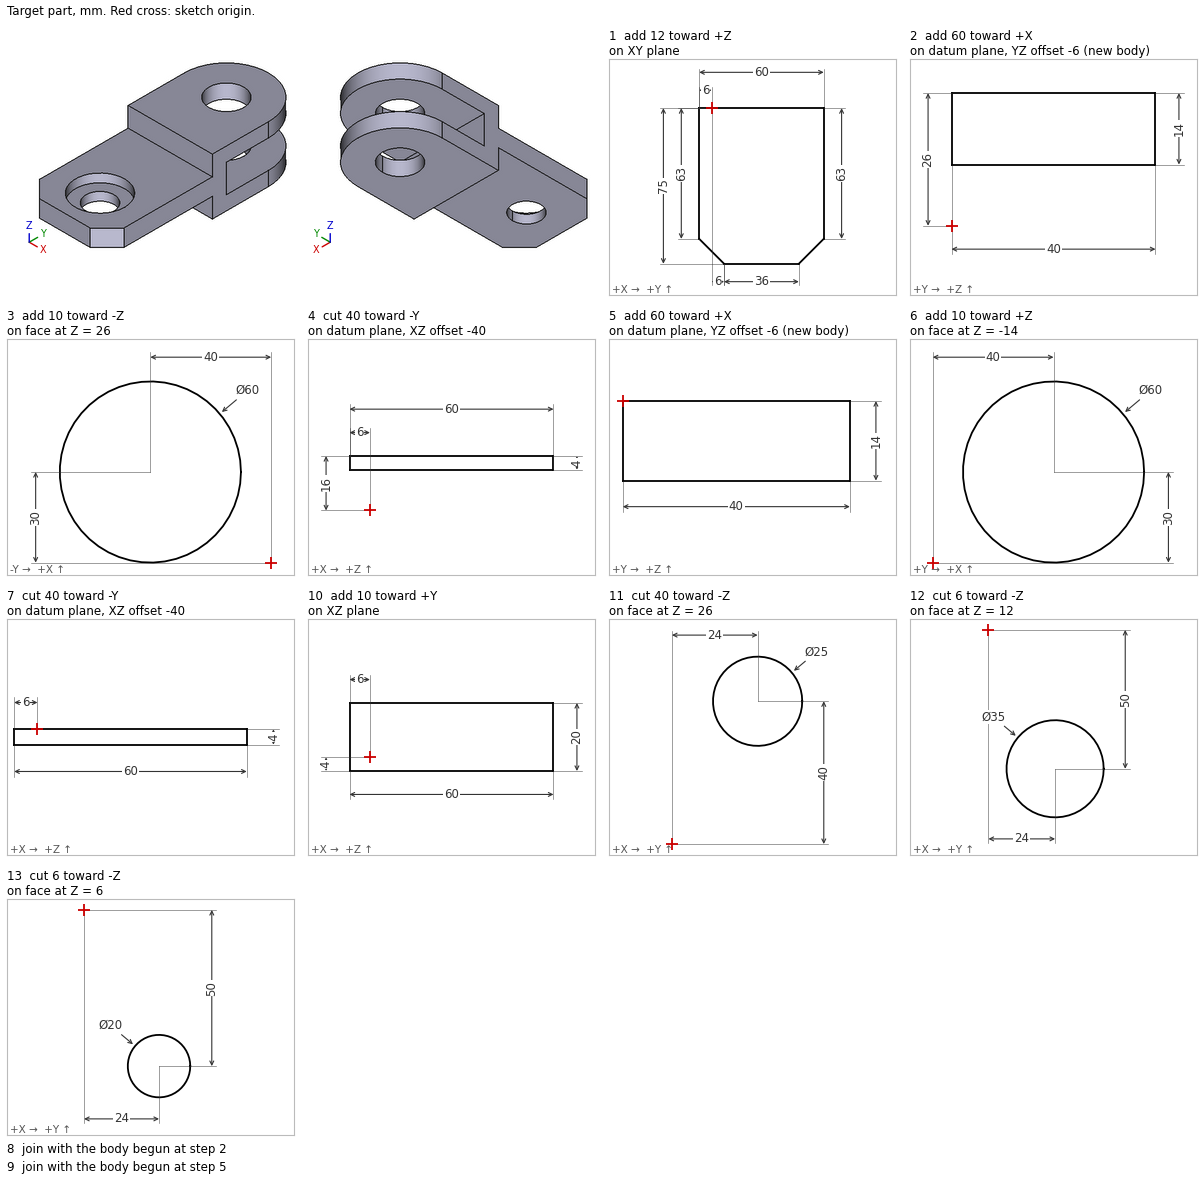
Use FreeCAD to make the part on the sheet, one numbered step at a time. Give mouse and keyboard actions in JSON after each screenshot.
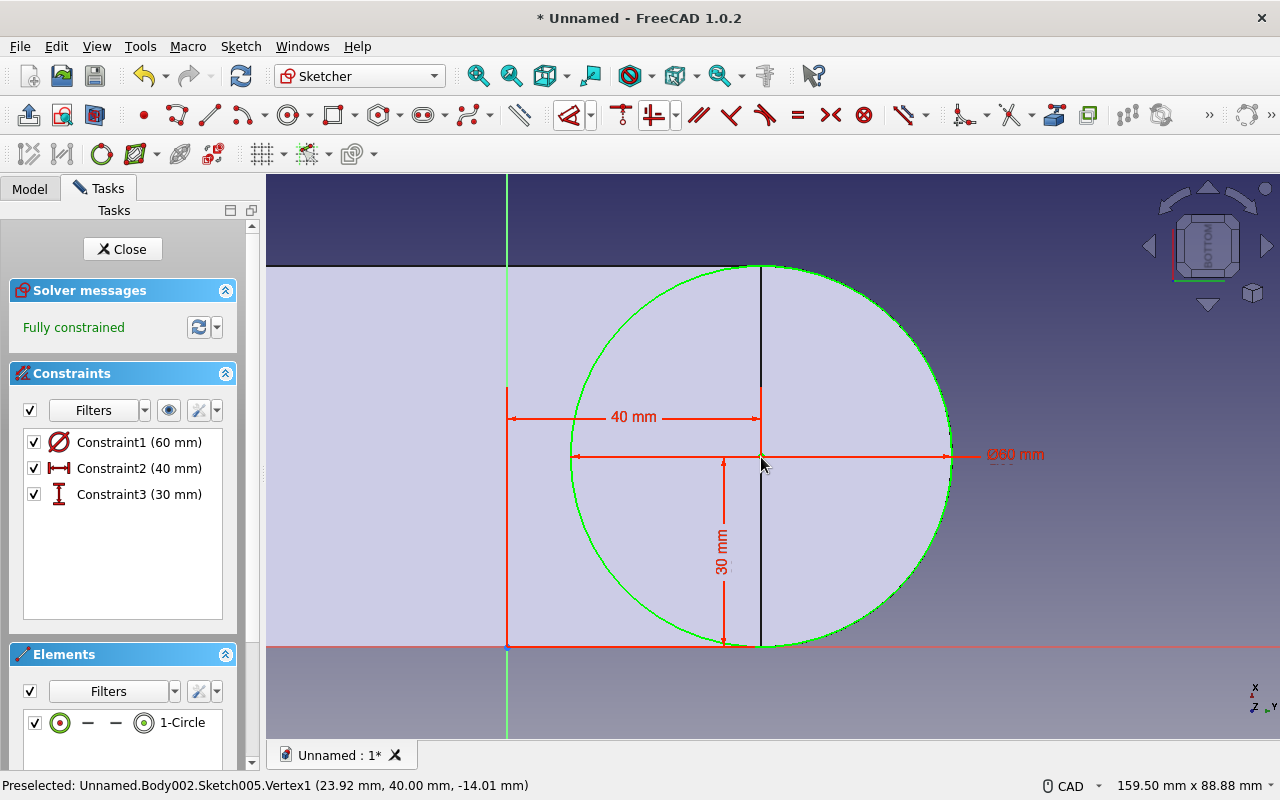
{"action": "left_click", "coordinate": [123, 249]}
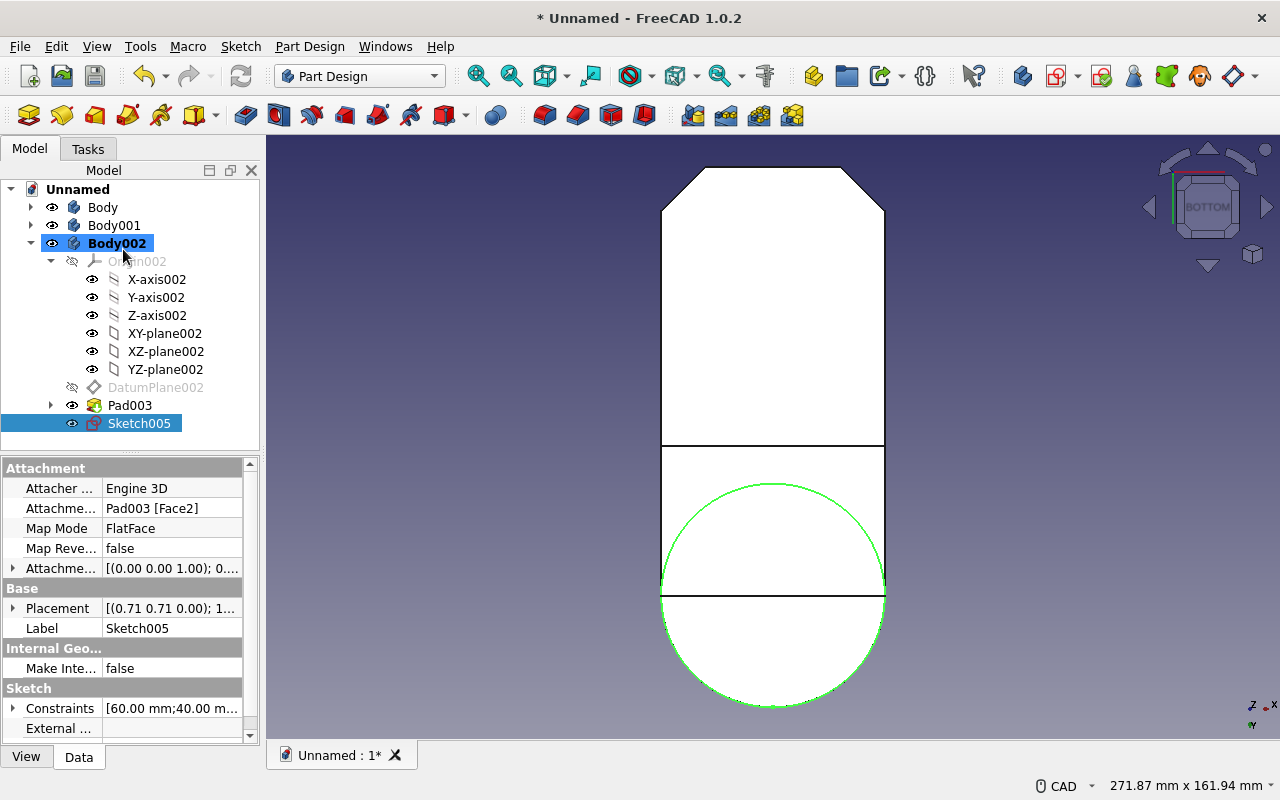
{"action": "left_click", "coordinate": [29, 116]}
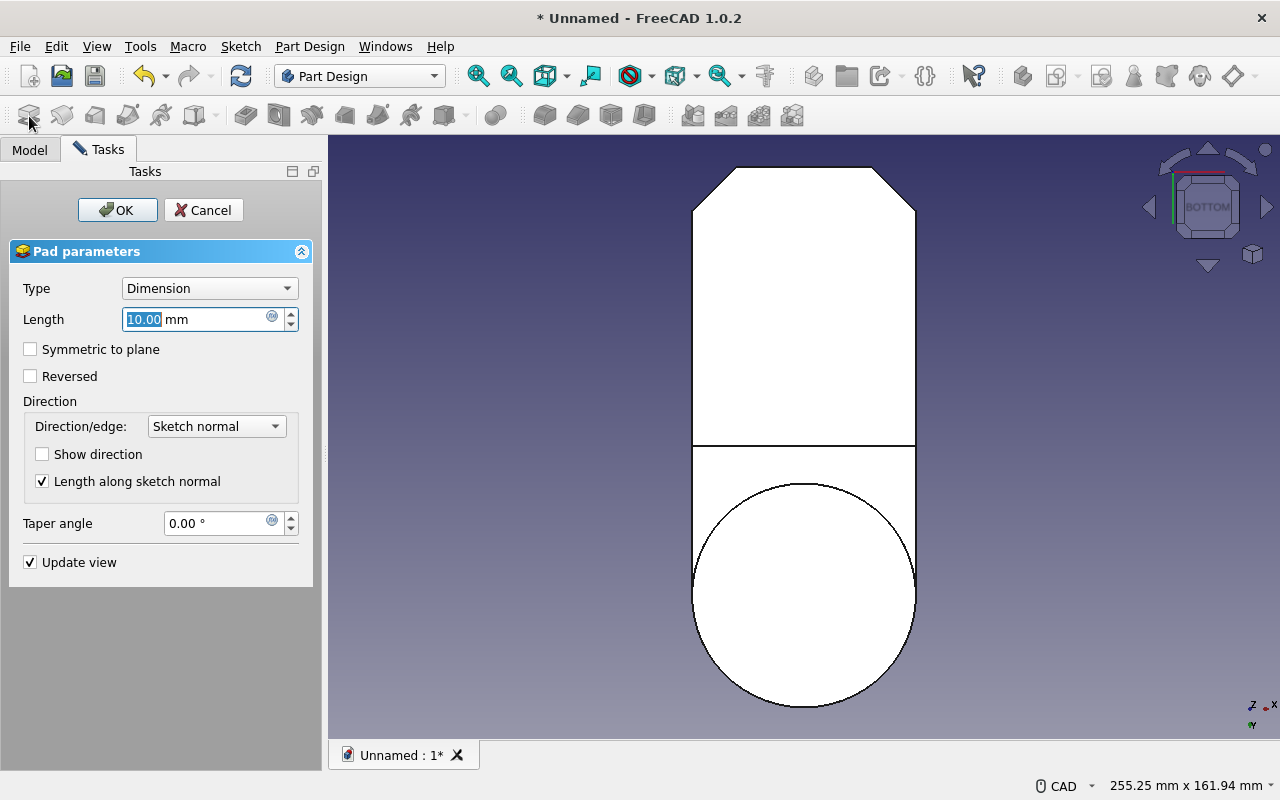
{"action": "type", "text": "10"}
{"action": "key", "text": "Tab"}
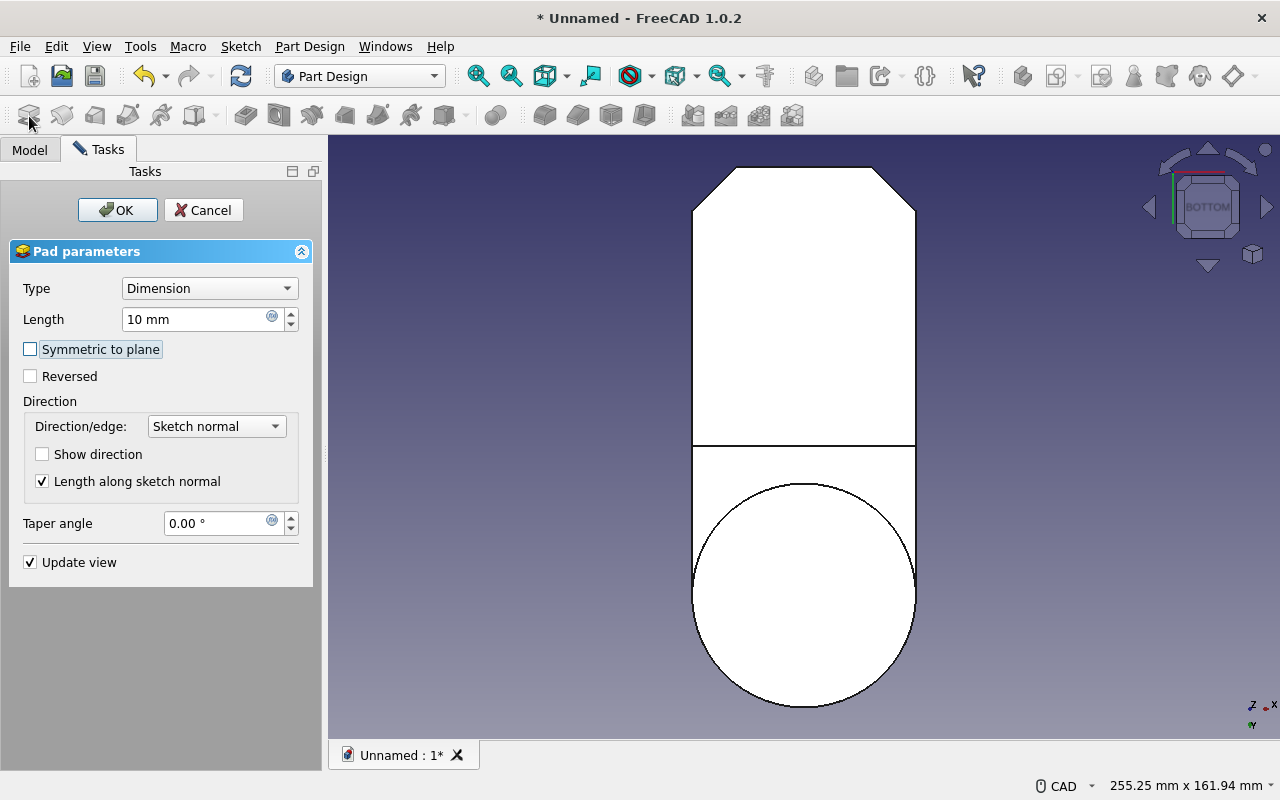
{"action": "left_click", "coordinate": [31, 376]}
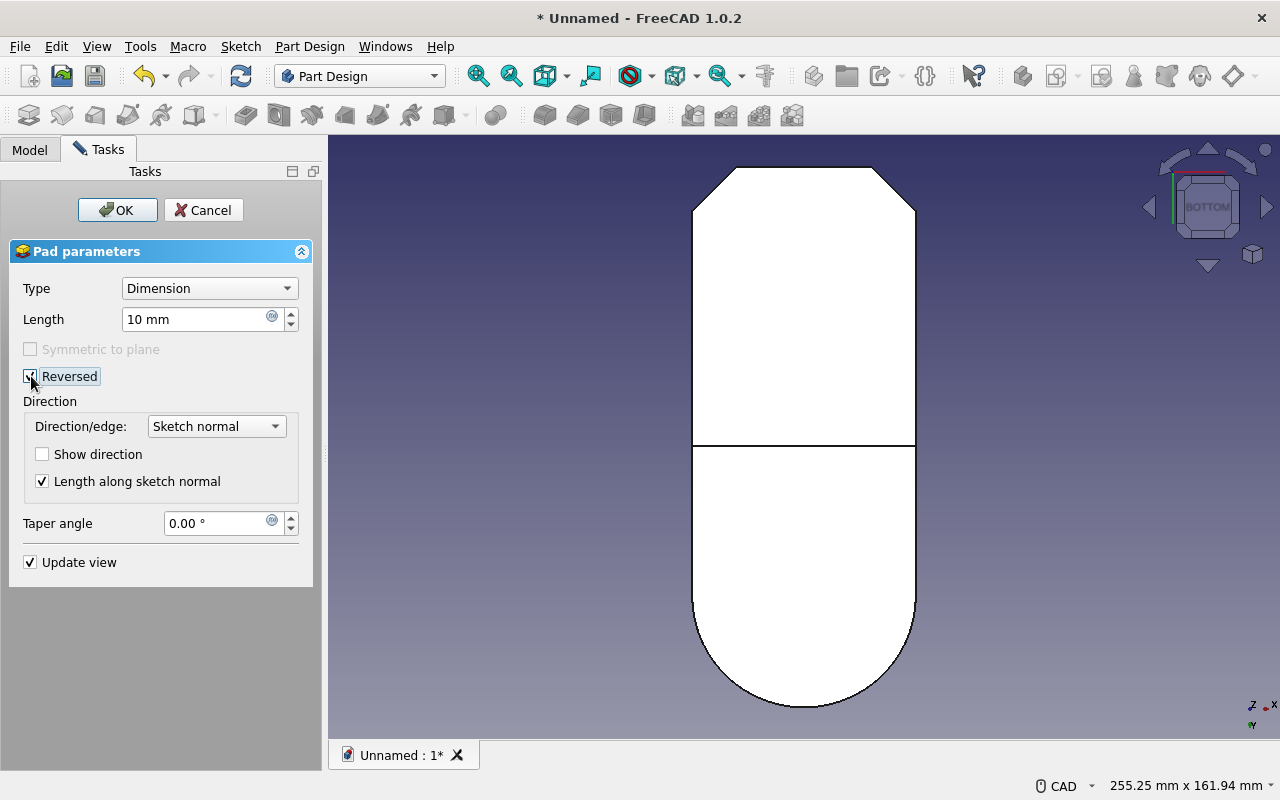
{"action": "left_click", "coordinate": [118, 210]}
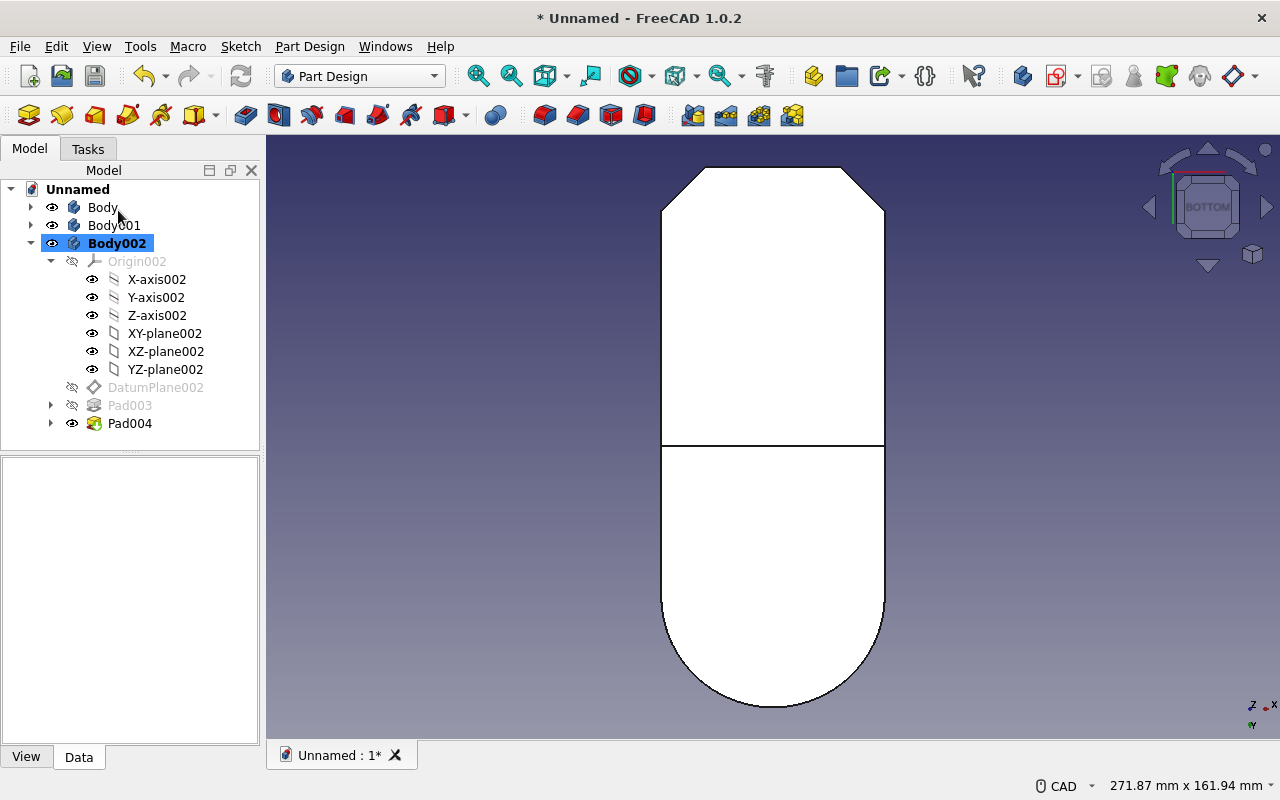
{"action": "left_click", "coordinate": [479, 76]}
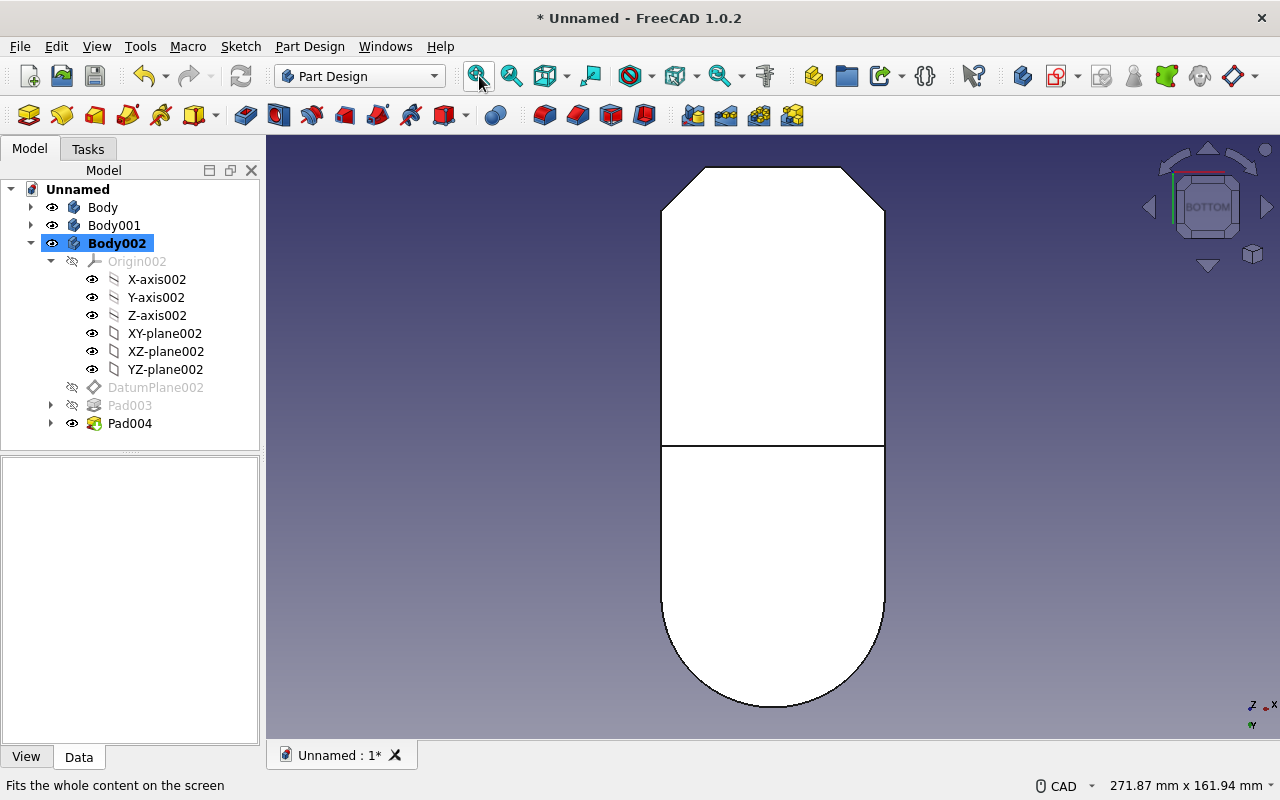
{"action": "key", "text": "4"}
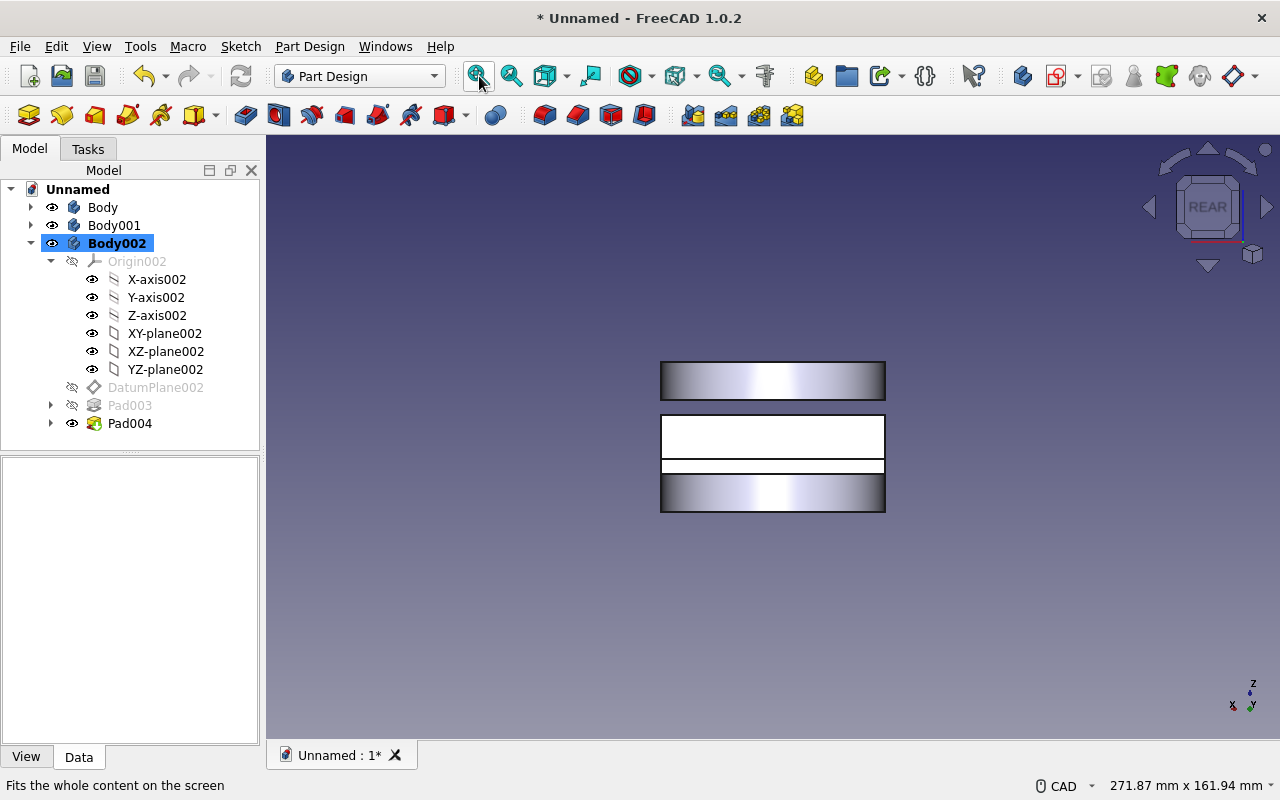
{"action": "key", "text": "v f"}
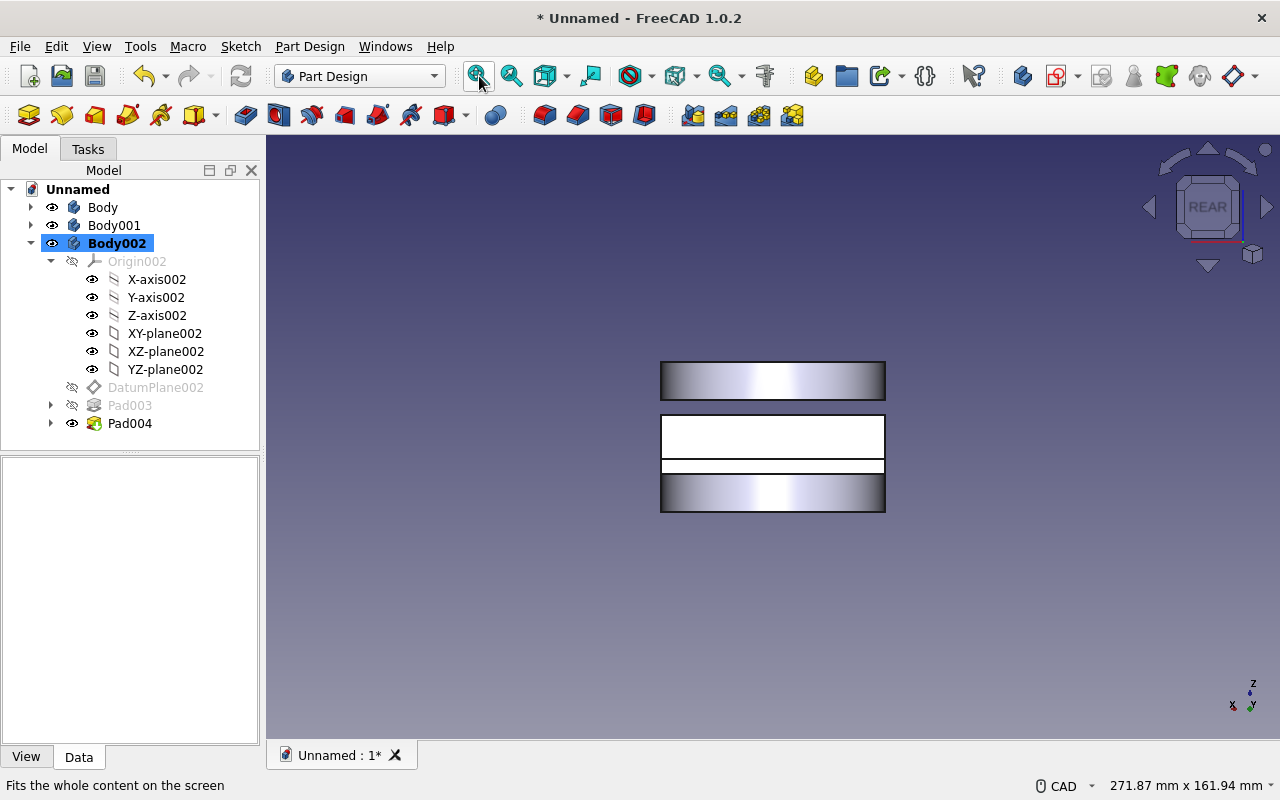
{"action": "key", "text": "5"}